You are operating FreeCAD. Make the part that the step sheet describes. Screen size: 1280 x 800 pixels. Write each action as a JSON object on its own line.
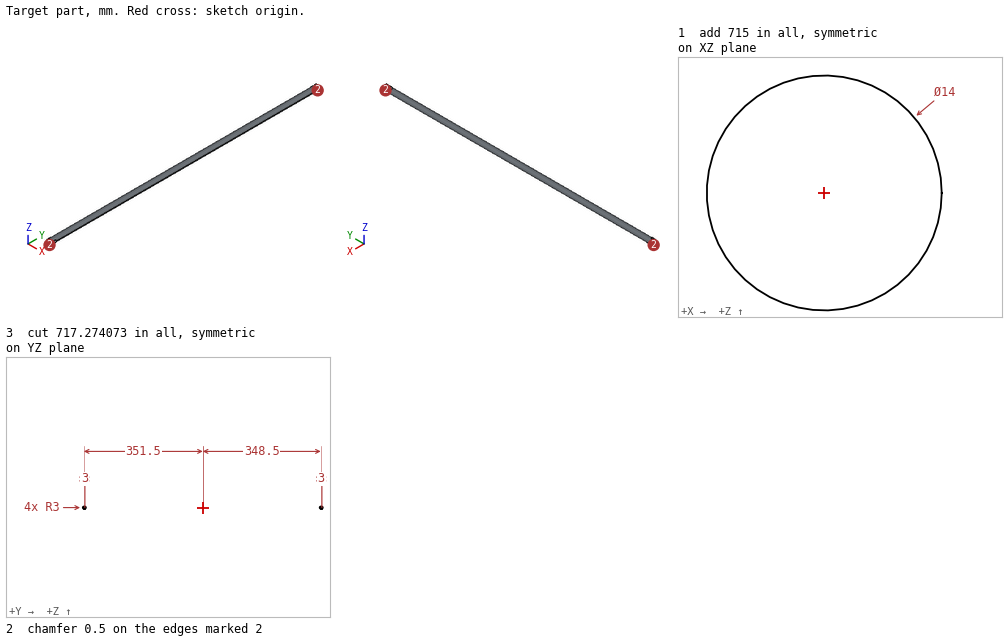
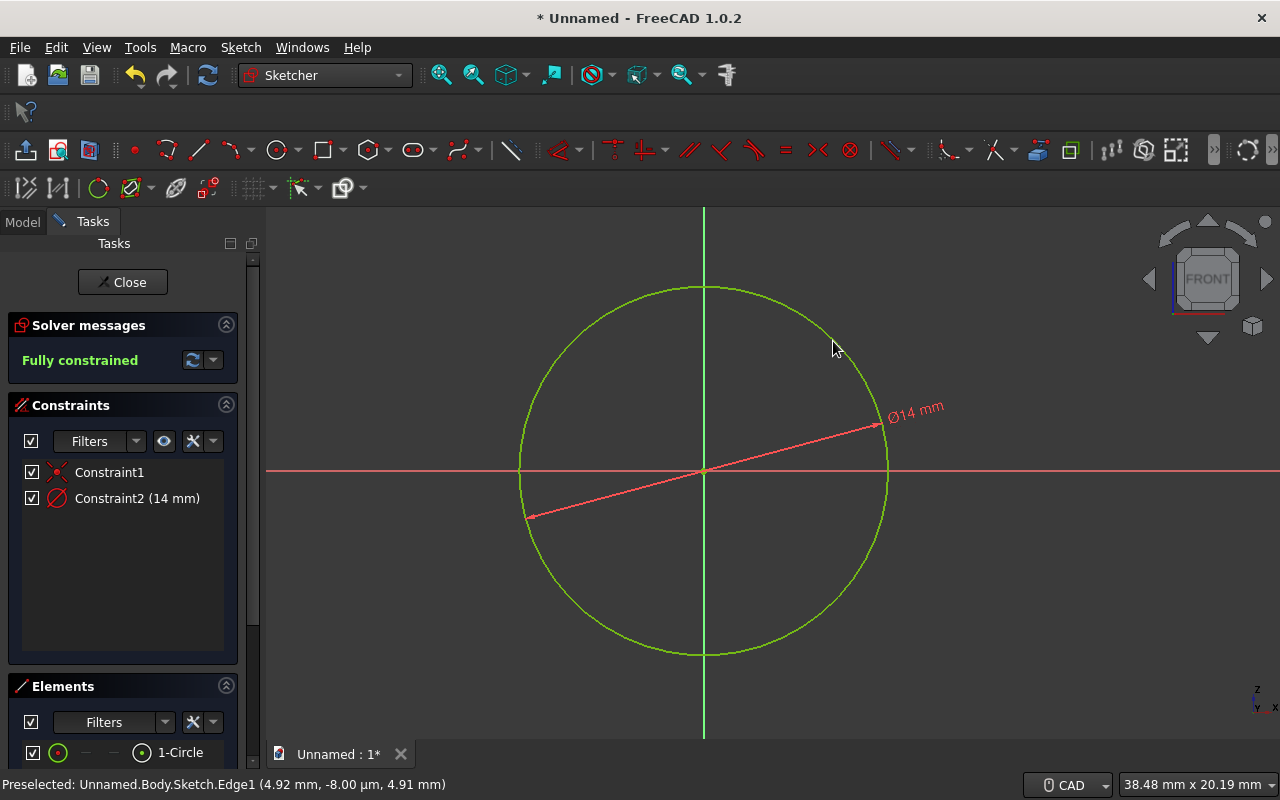
{"action": "left_click", "coordinate": [123, 282]}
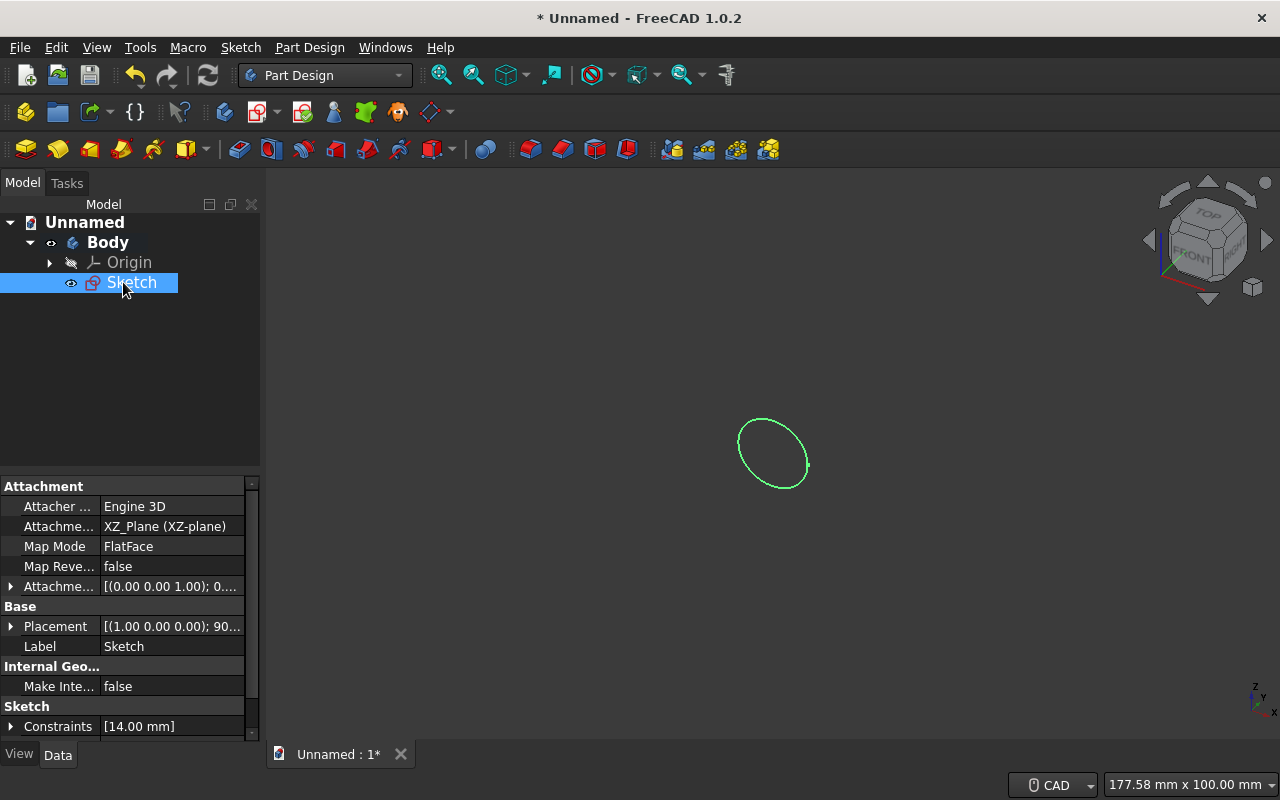
{"action": "left_click", "coordinate": [26, 150]}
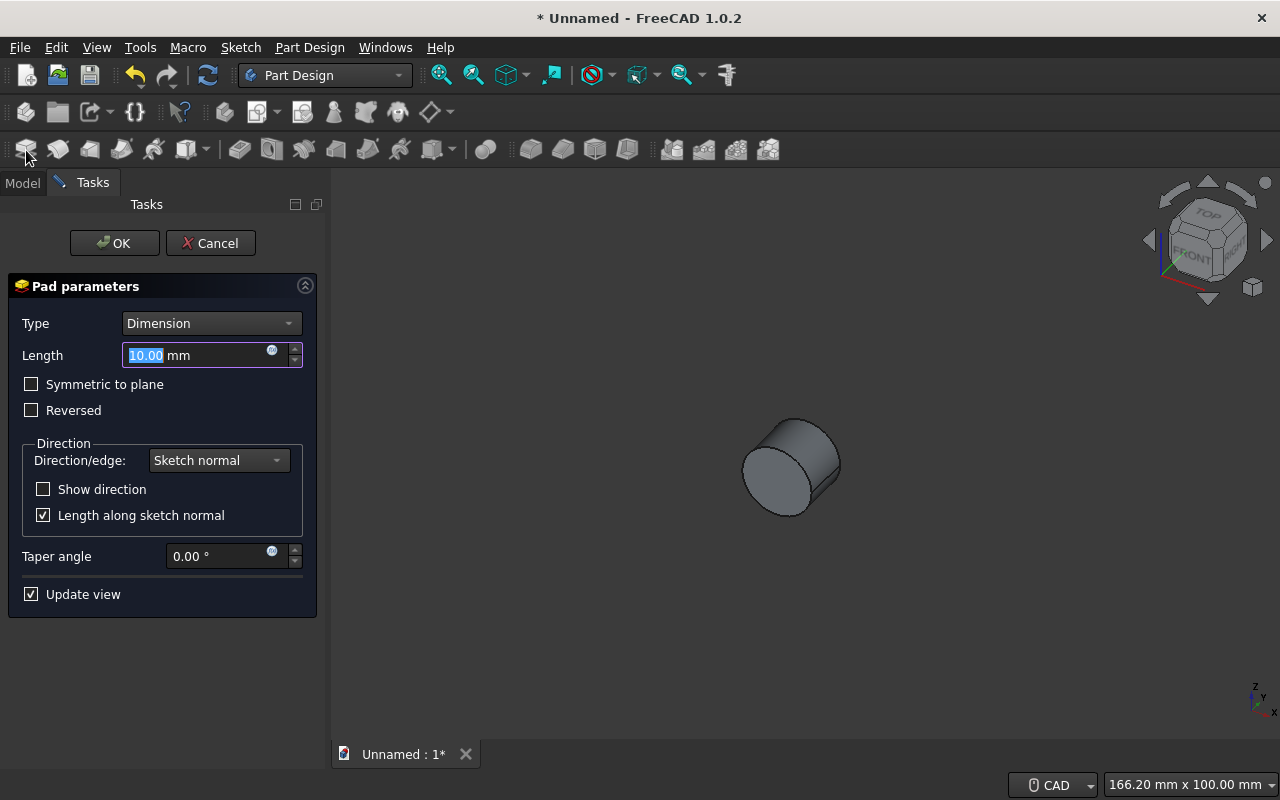
{"action": "type", "text": "715"}
{"action": "key", "text": "Tab"}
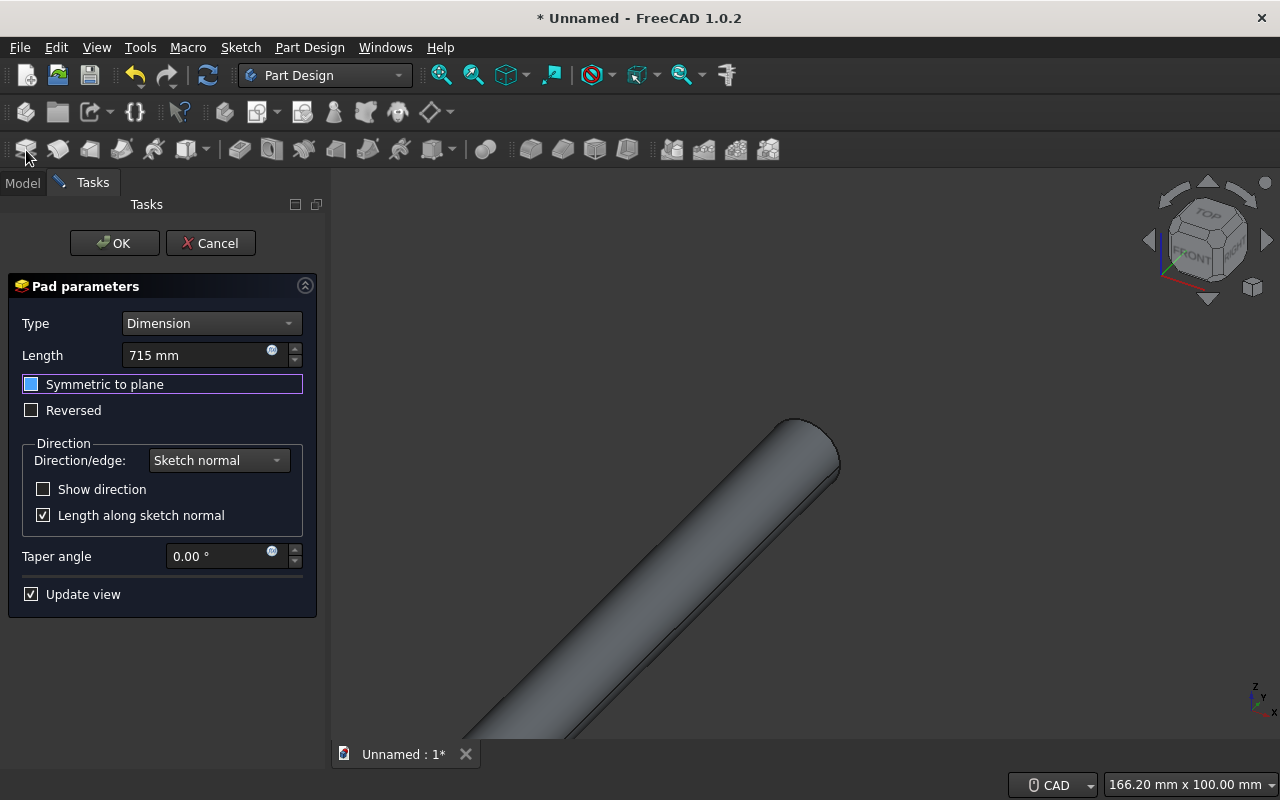
{"action": "left_click", "coordinate": [30, 384]}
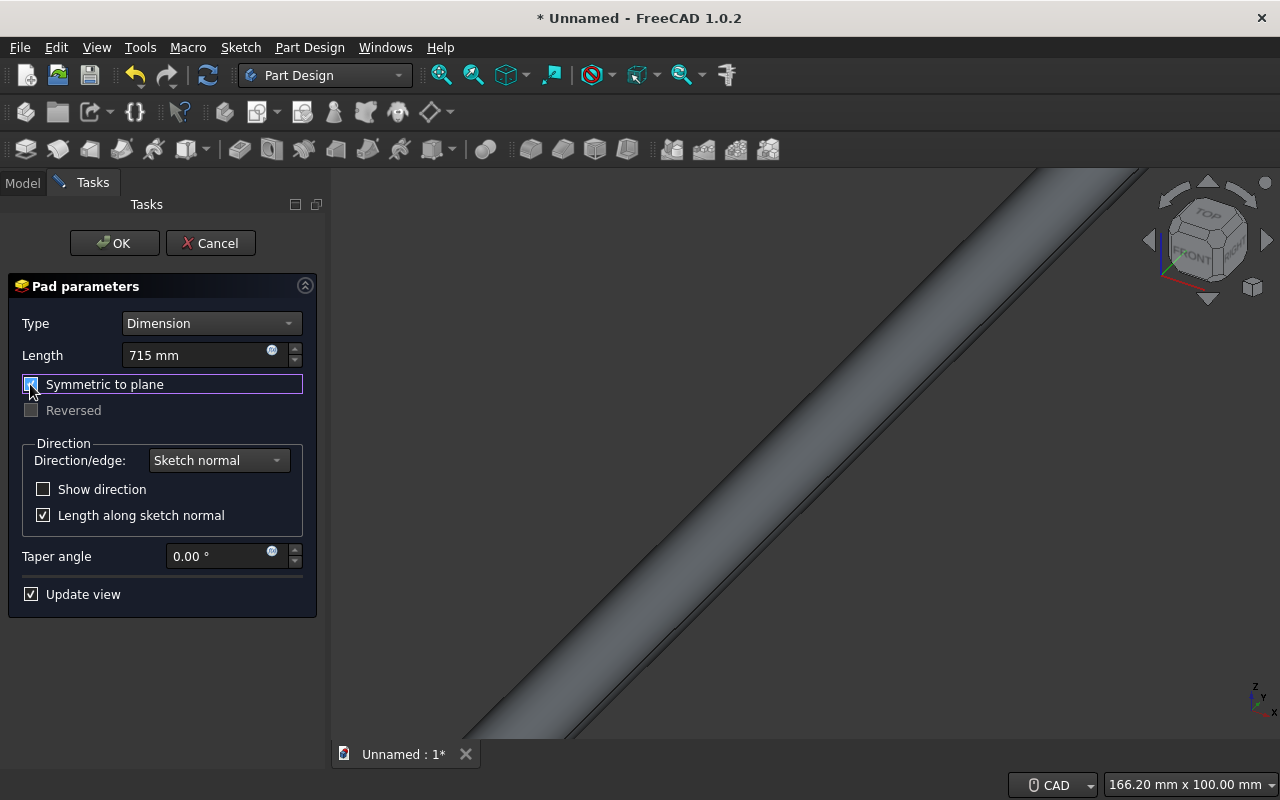
{"action": "left_click", "coordinate": [115, 243]}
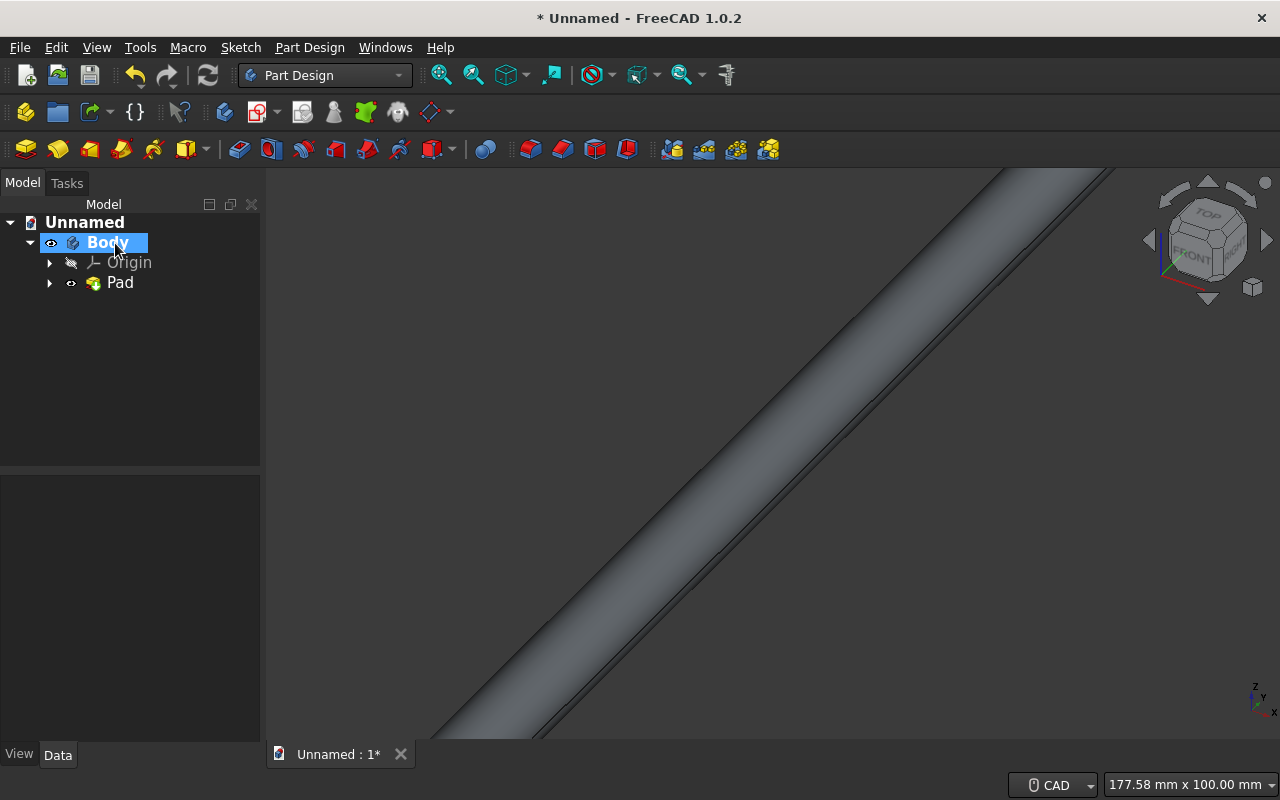
{"action": "left_click", "coordinate": [442, 76]}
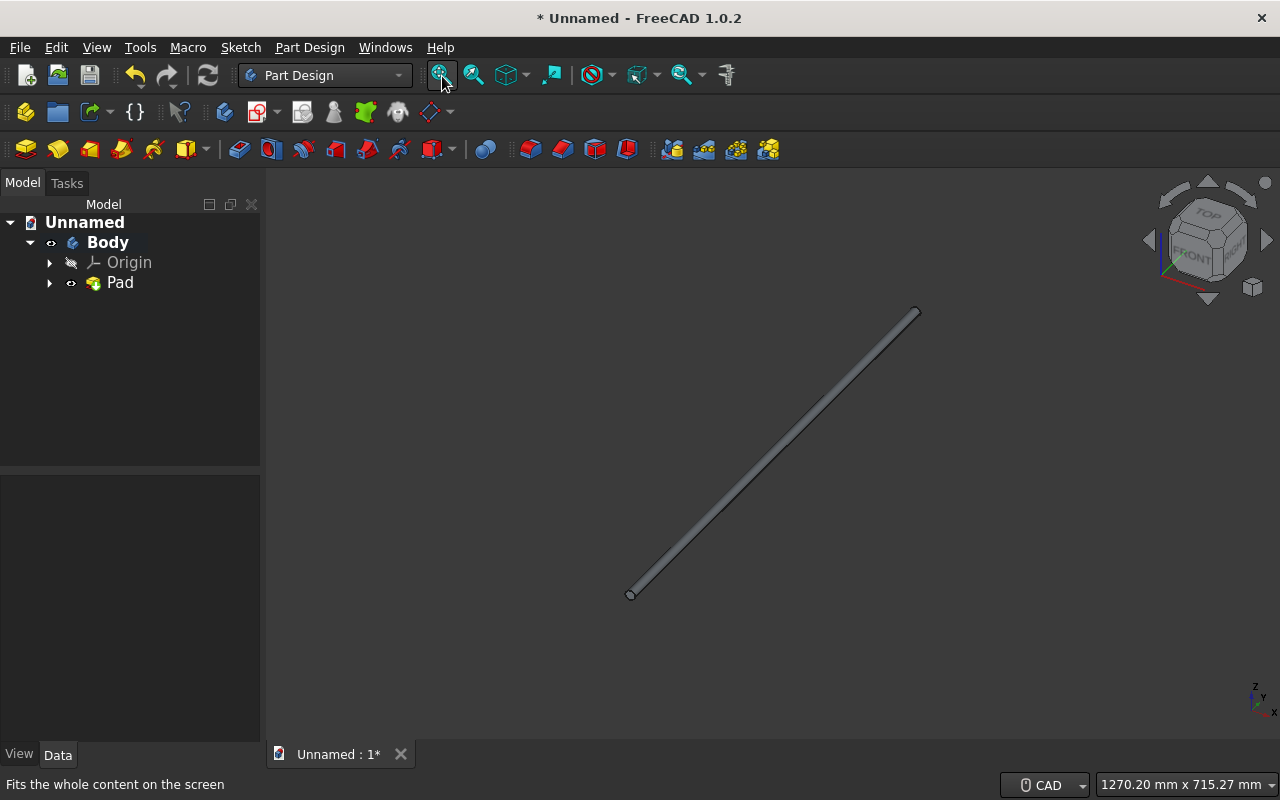
{"action": "left_click", "coordinate": [625, 593]}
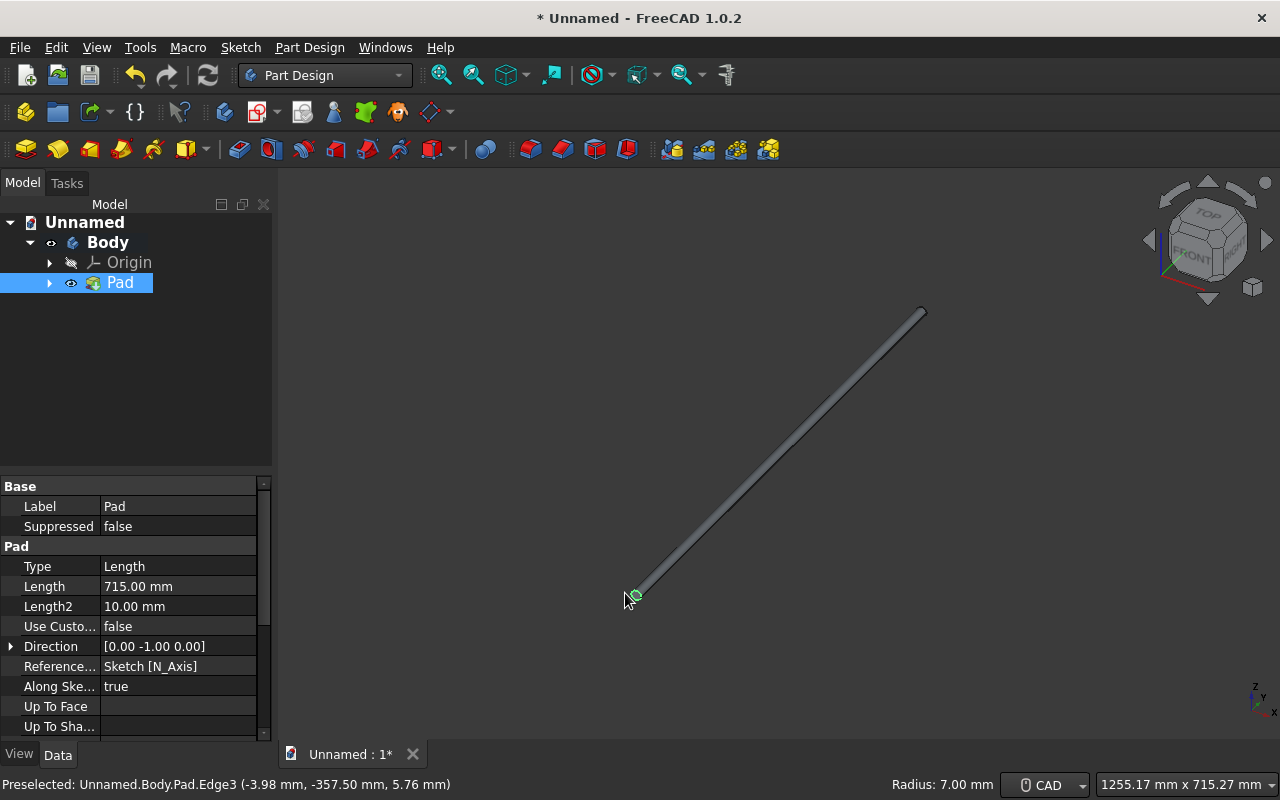
{"action": "key", "text": "0"}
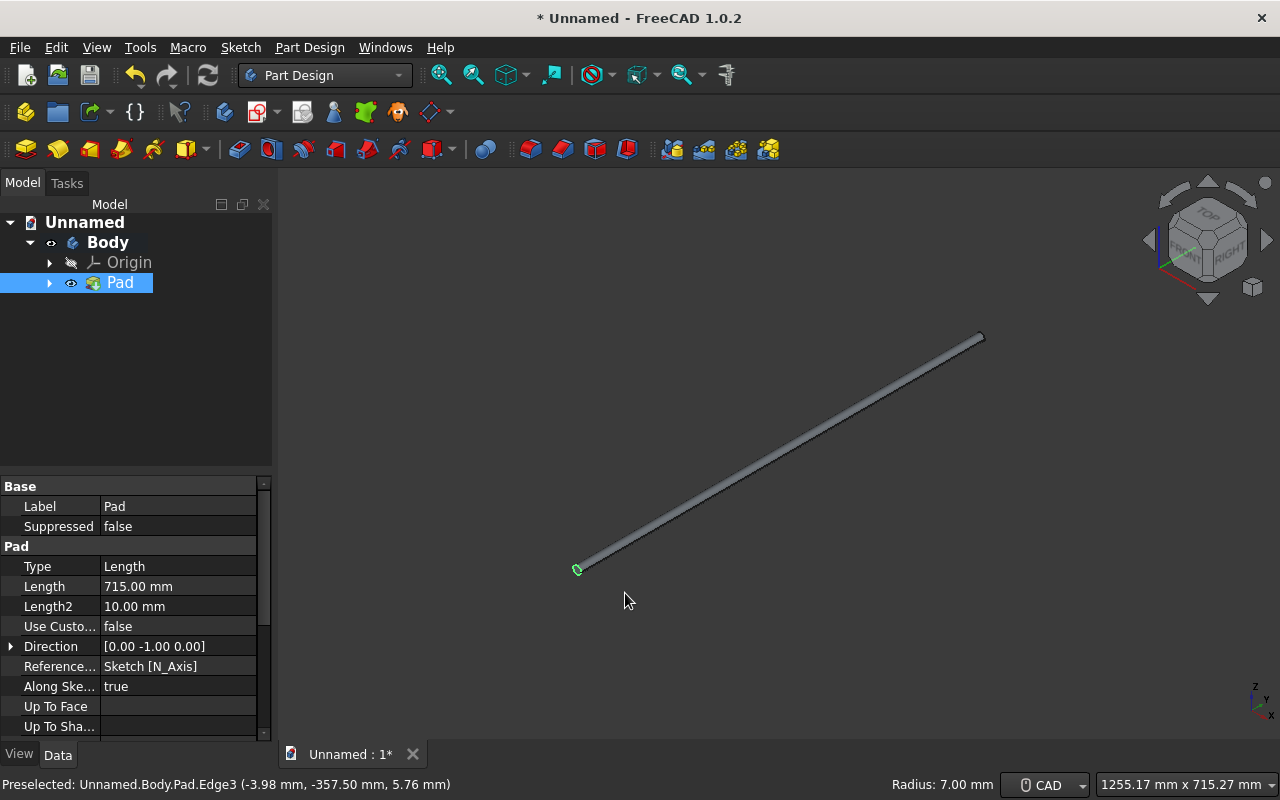
{"action": "left_click", "coordinate": [442, 76]}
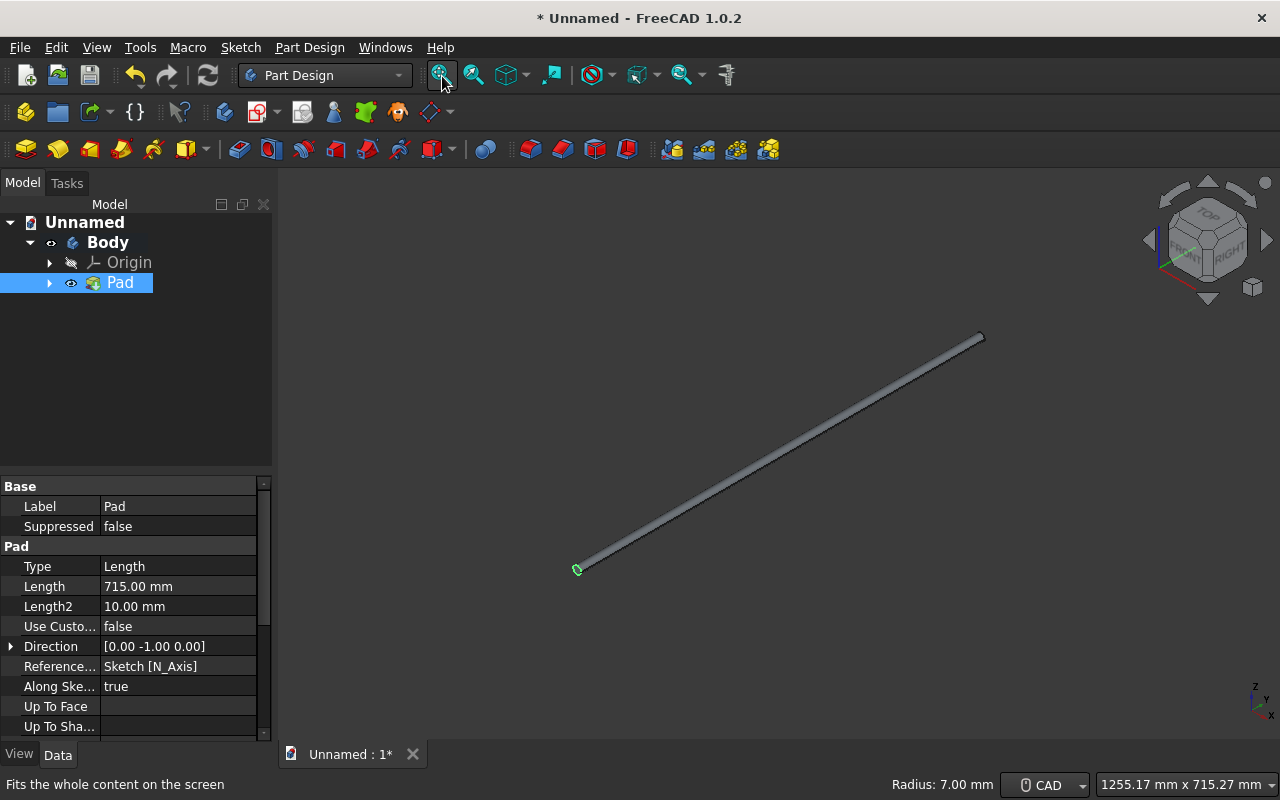
{"action": "left_click", "coordinate": [978, 331], "text": "ctrl"}